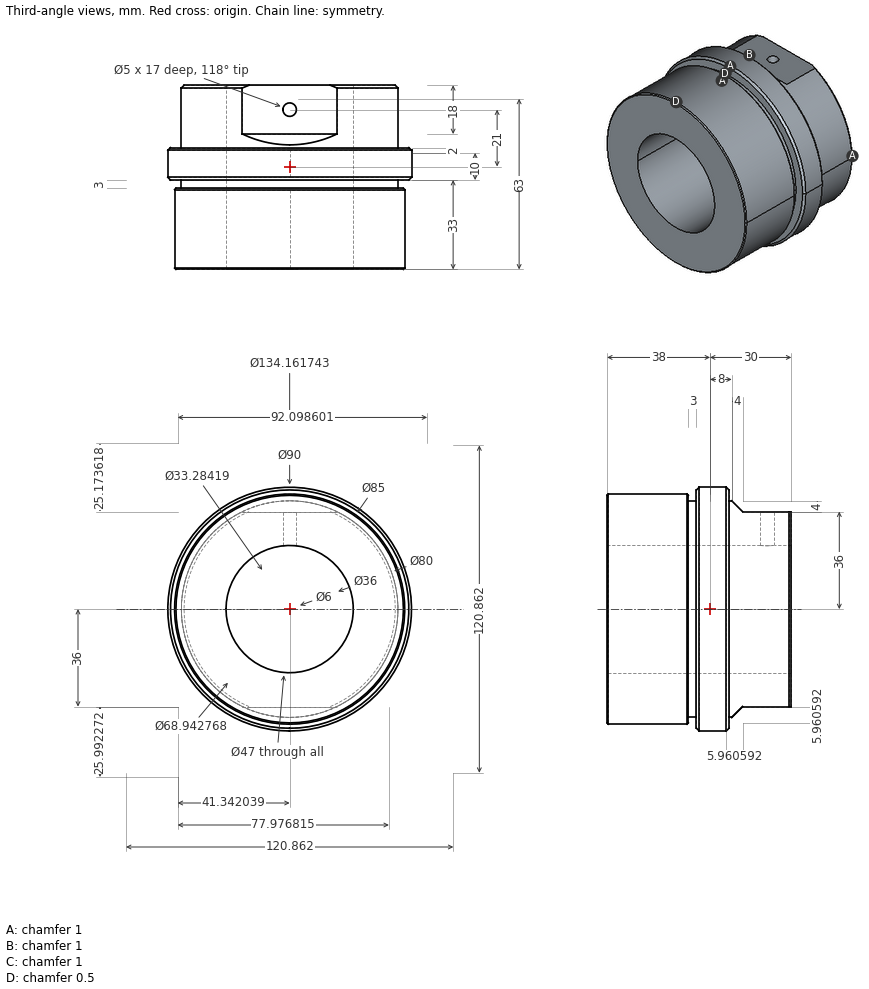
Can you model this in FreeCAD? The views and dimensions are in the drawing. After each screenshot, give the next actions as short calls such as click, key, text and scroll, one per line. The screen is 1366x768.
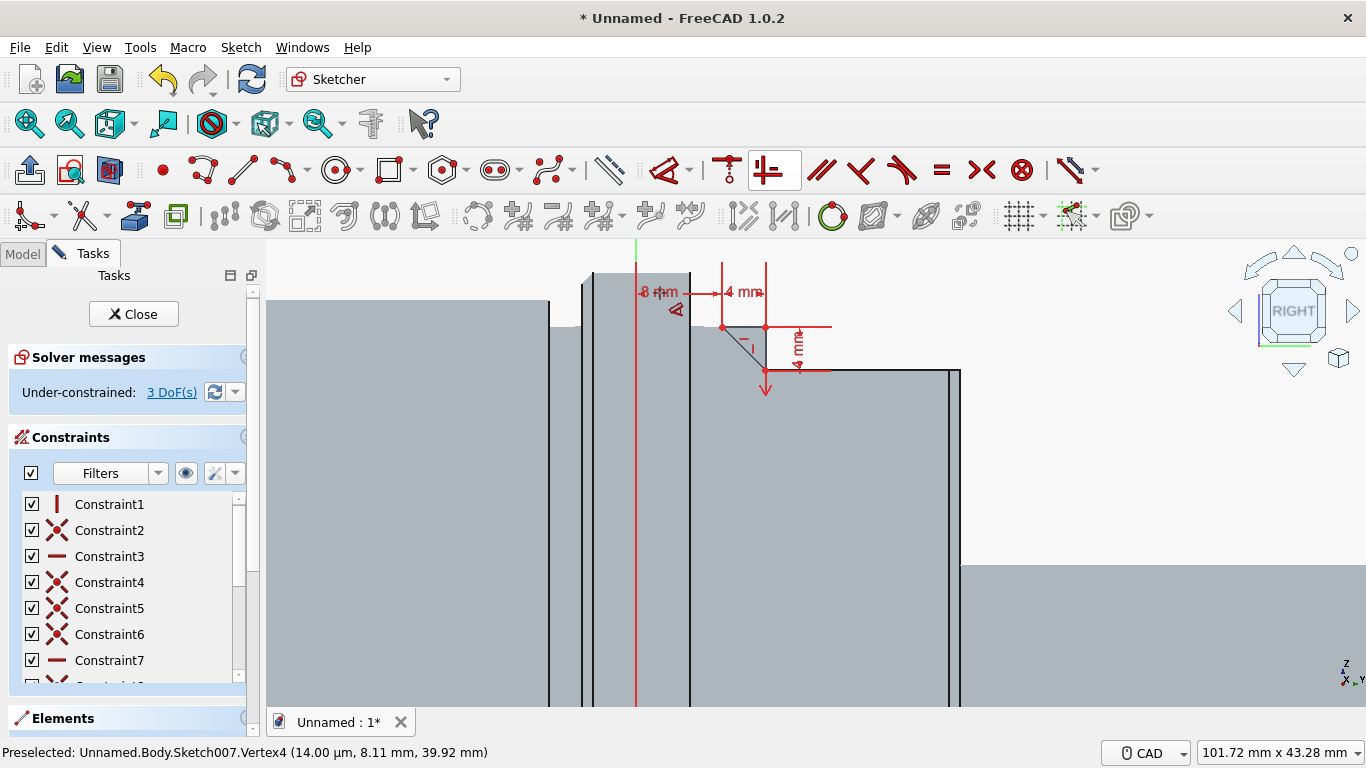
scroll(768, 345, down, 6)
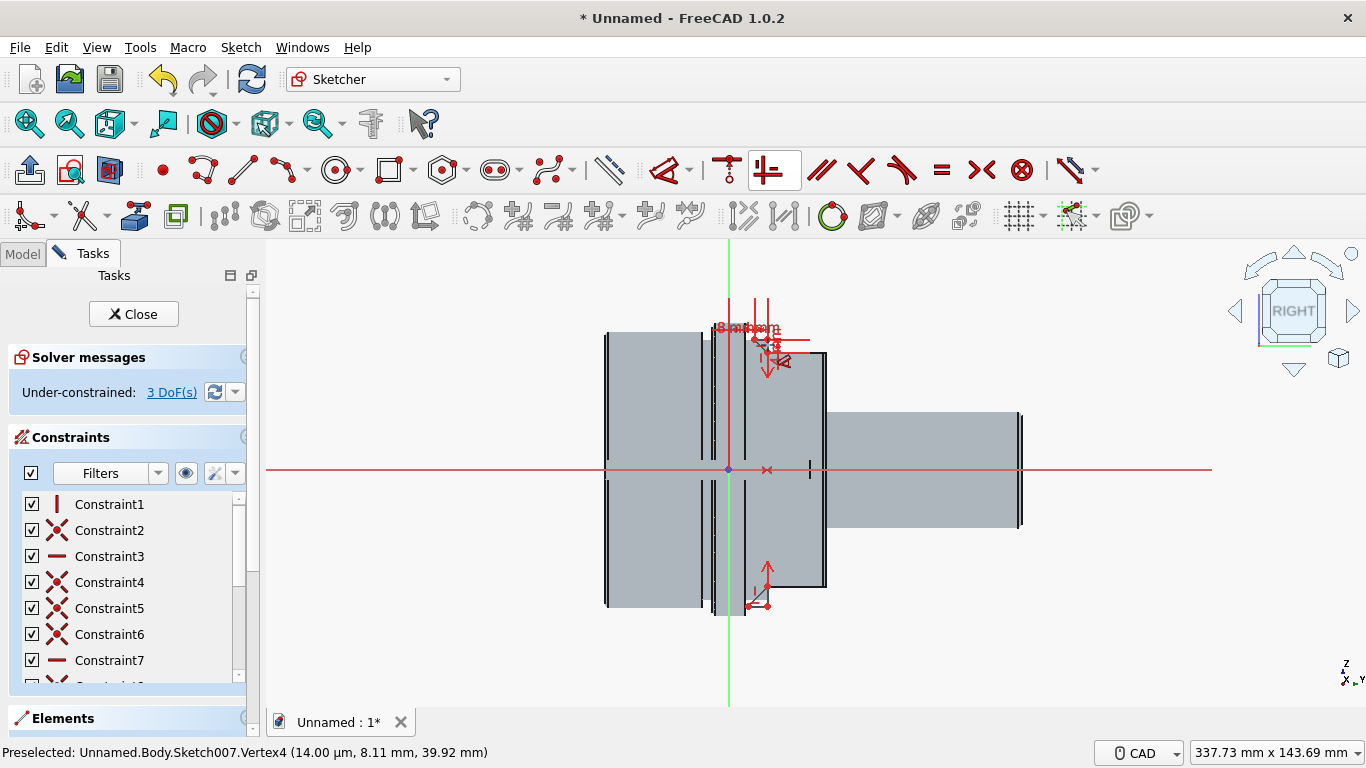
click(768, 353)
click(802, 411)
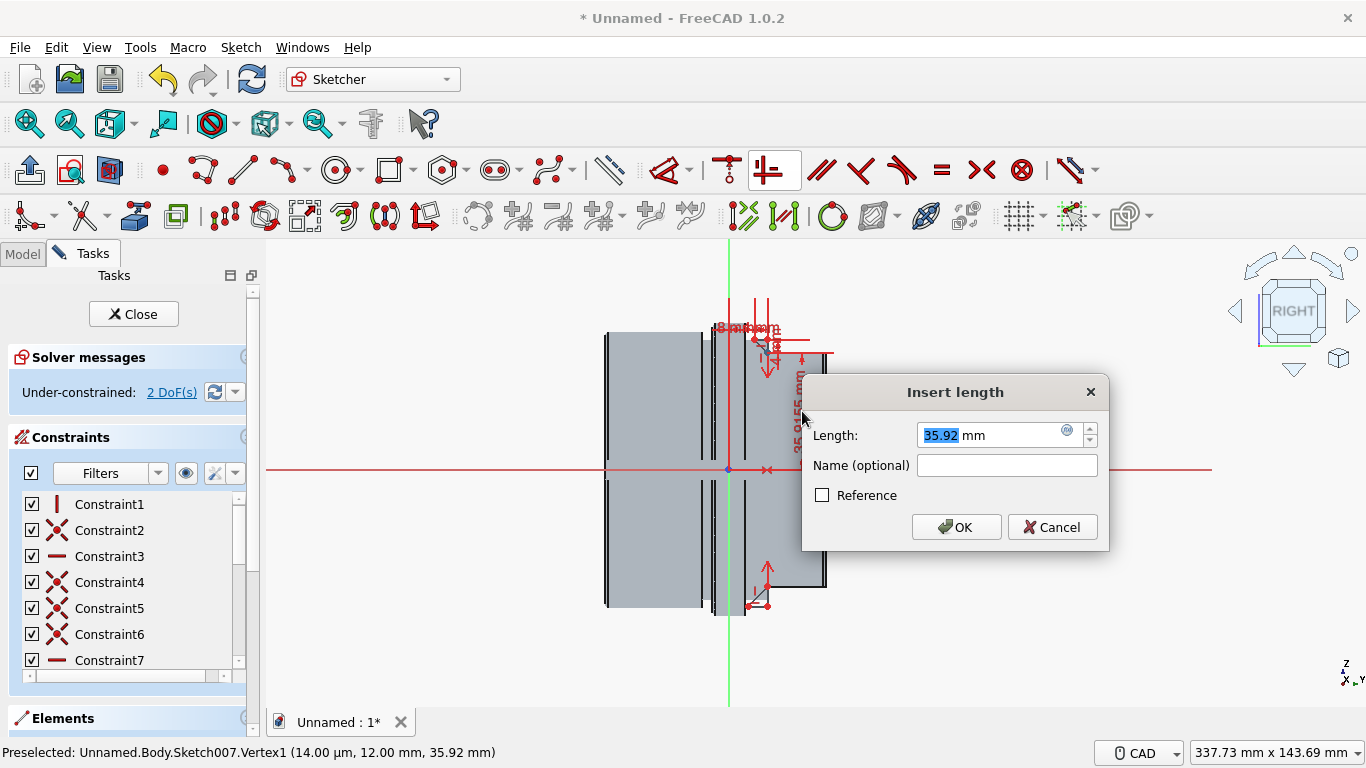
text(36)
key(Return)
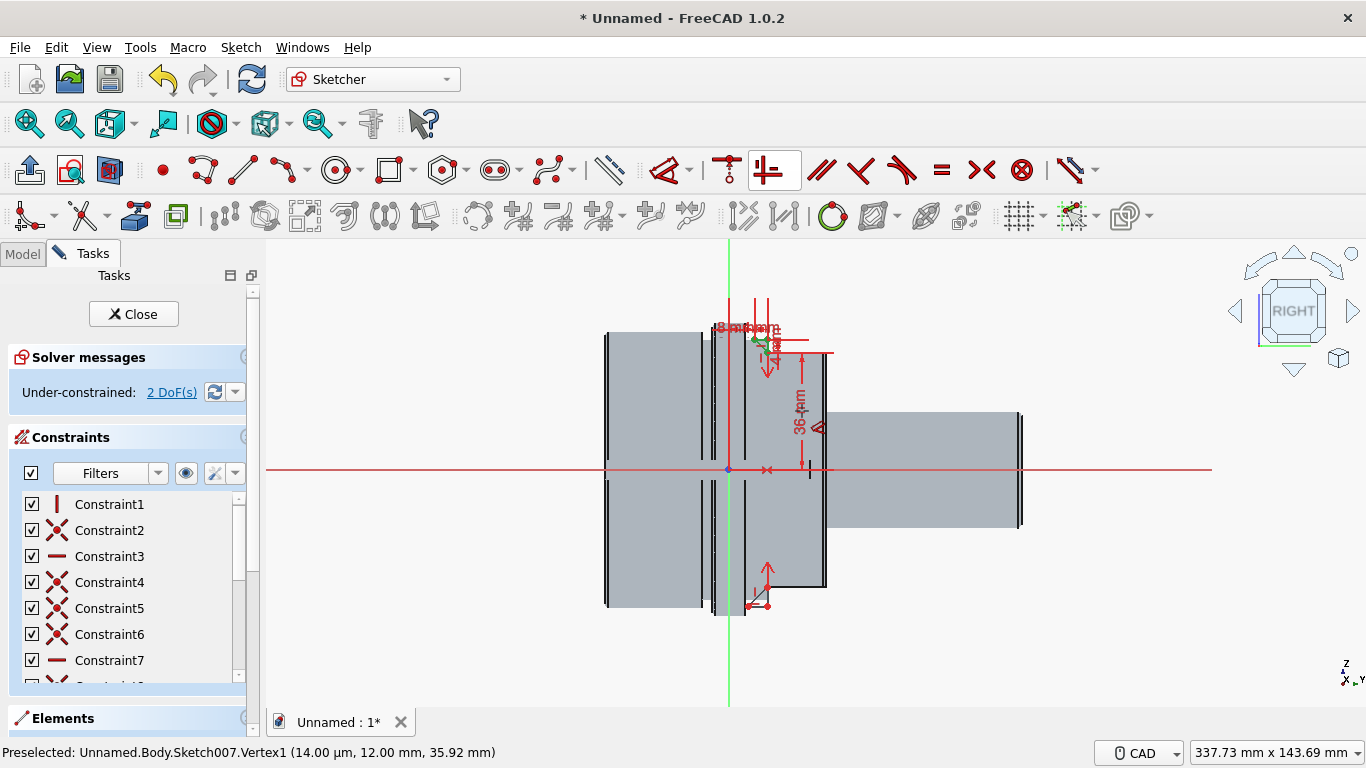
scroll(760, 607, up, 4)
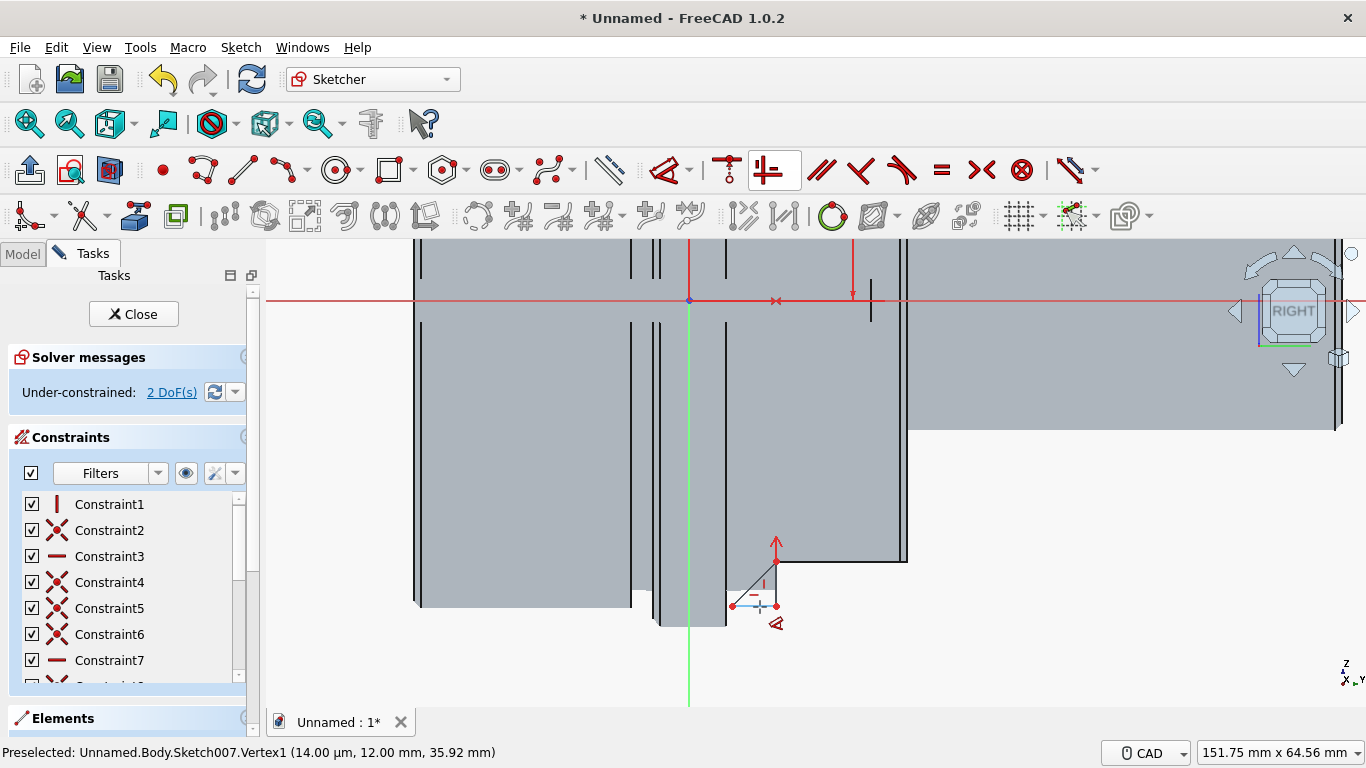
click(759, 606)
click(755, 640)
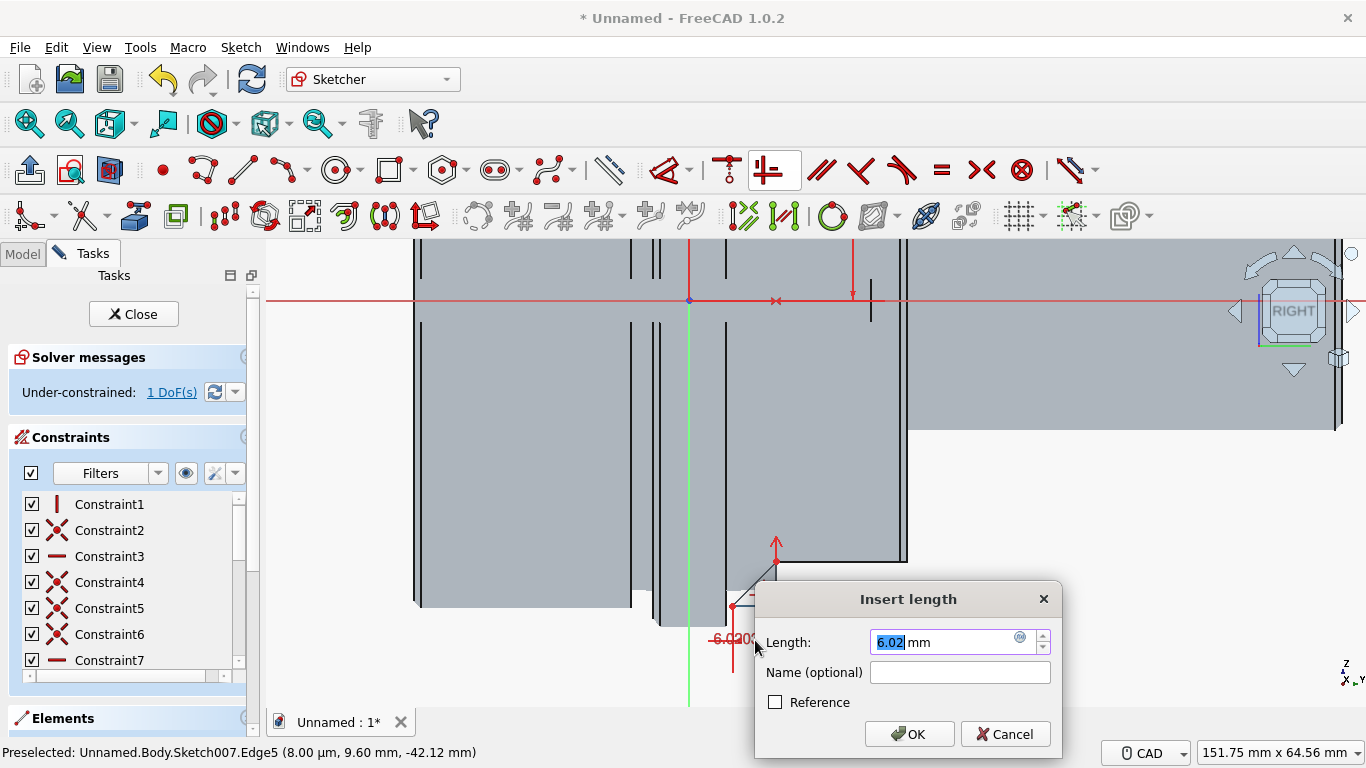
text(5.960592)
key(Return)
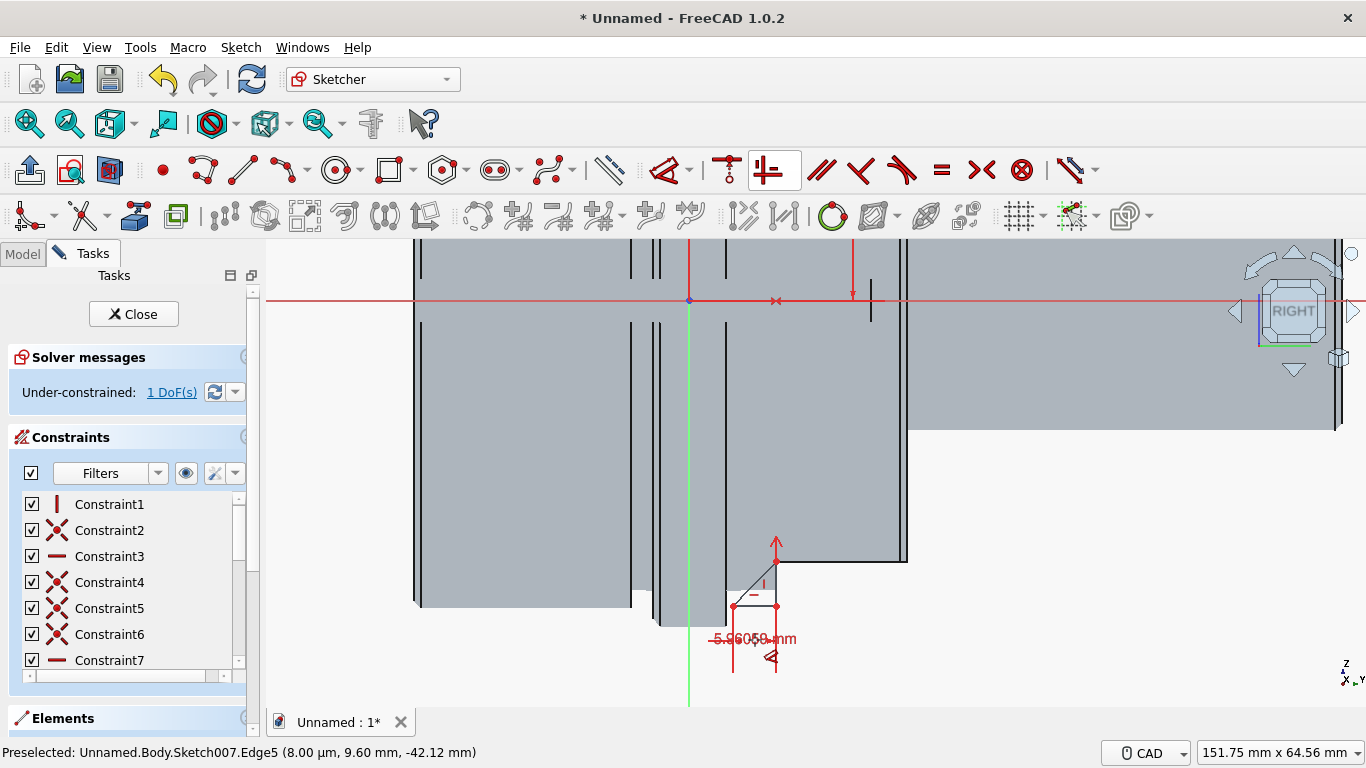
click(776, 593)
click(810, 584)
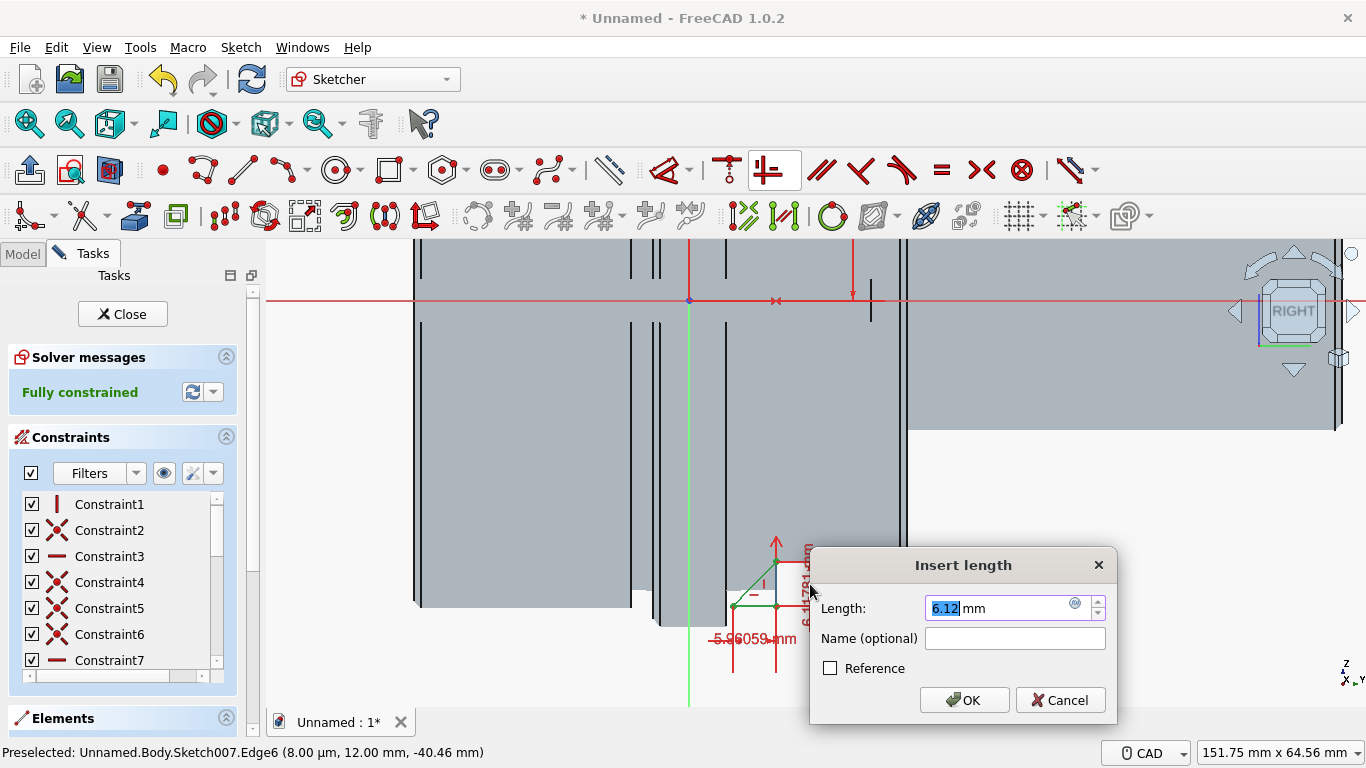
text(5.960592)
key(Return)
key(Escape)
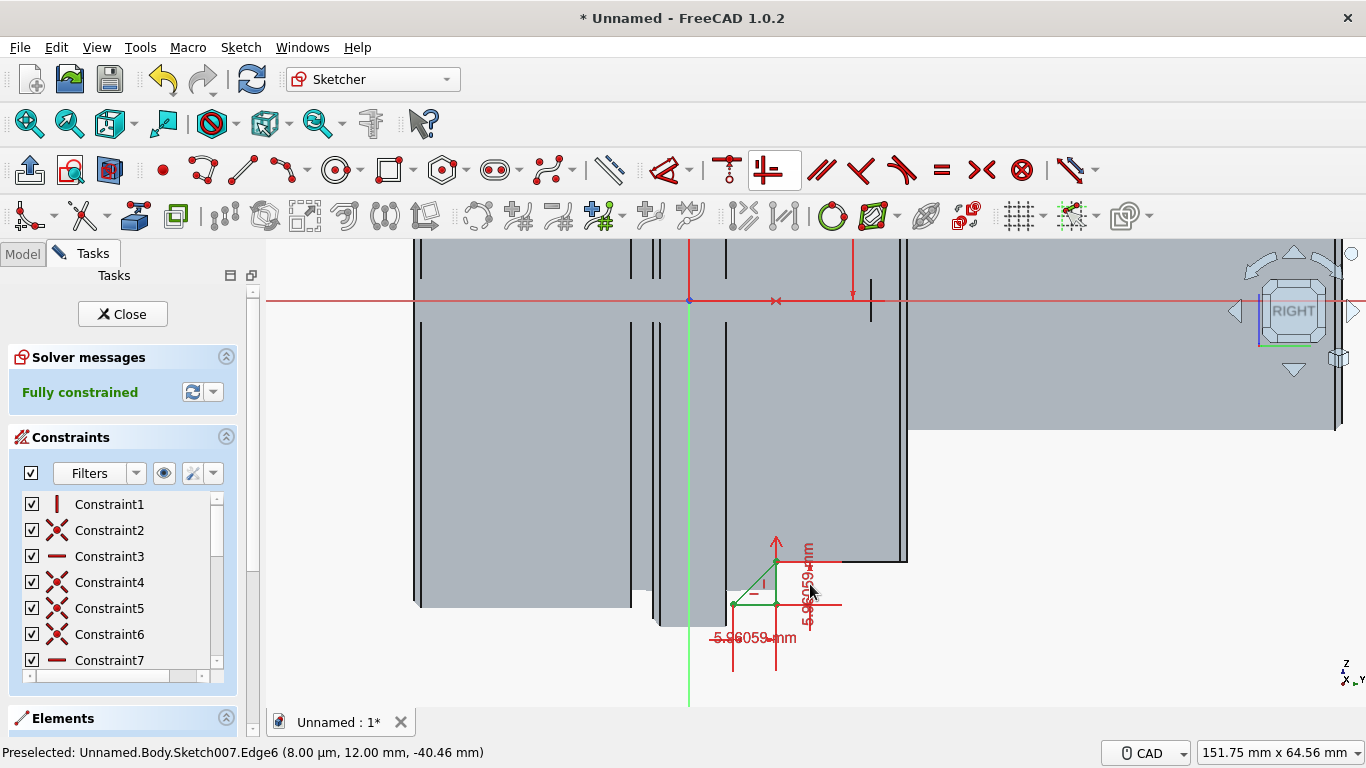
click(123, 314)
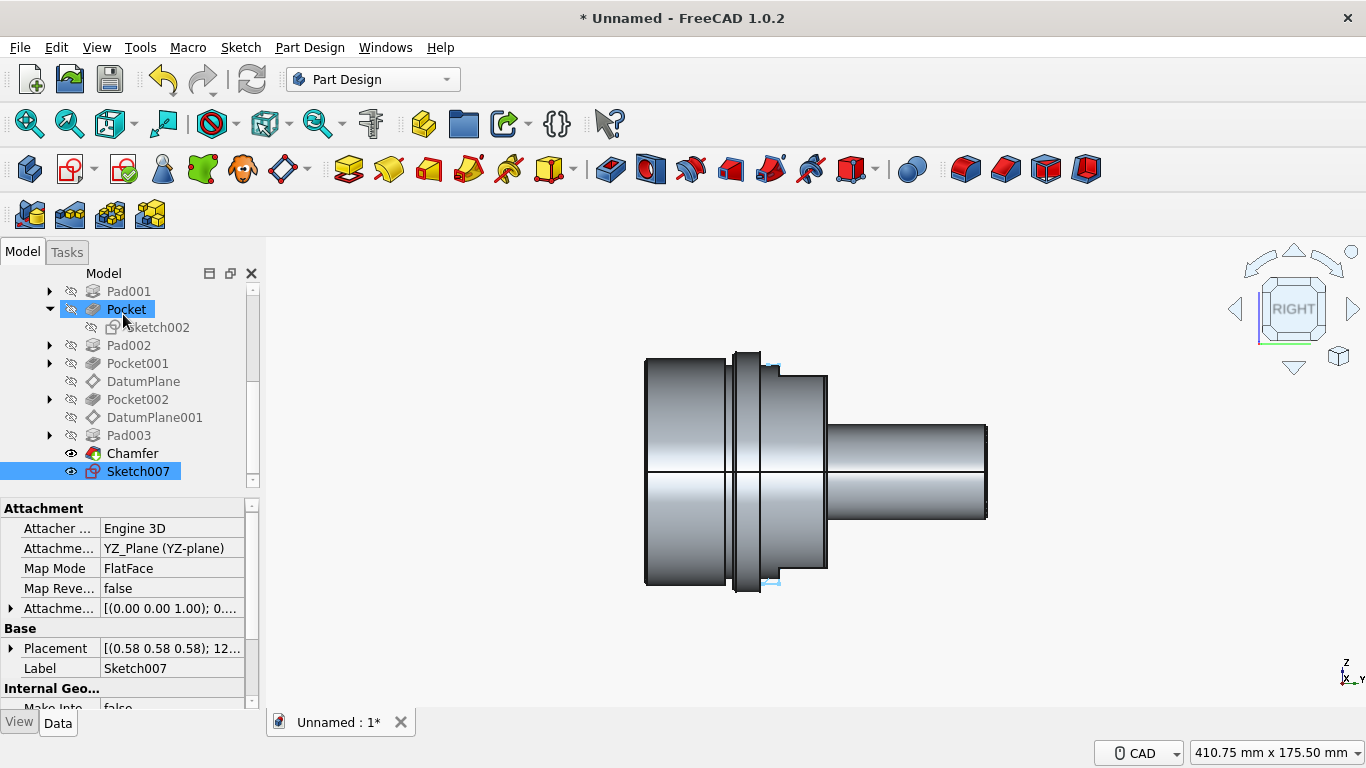
click(612, 170)